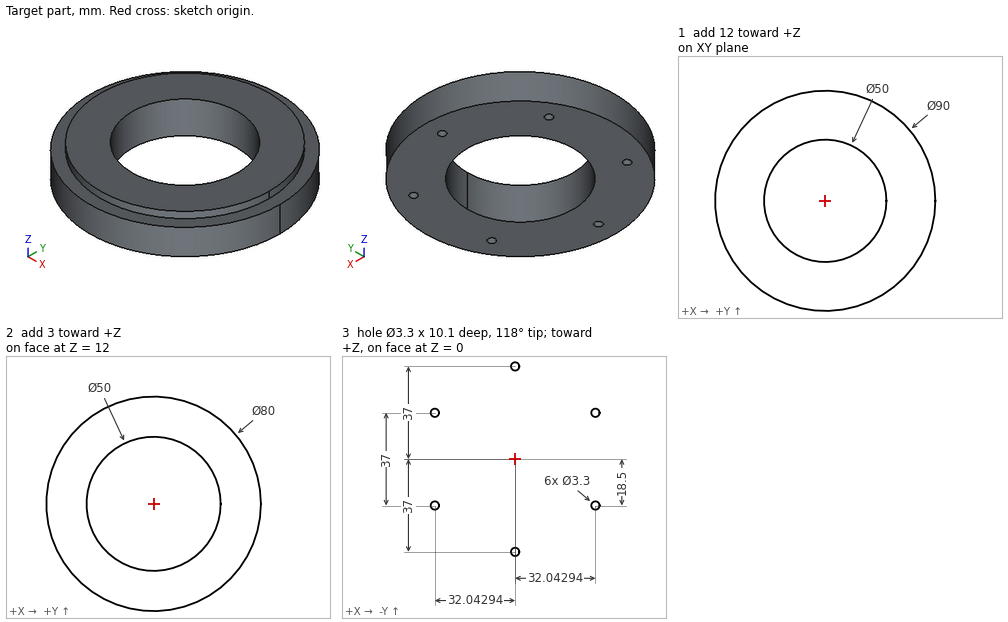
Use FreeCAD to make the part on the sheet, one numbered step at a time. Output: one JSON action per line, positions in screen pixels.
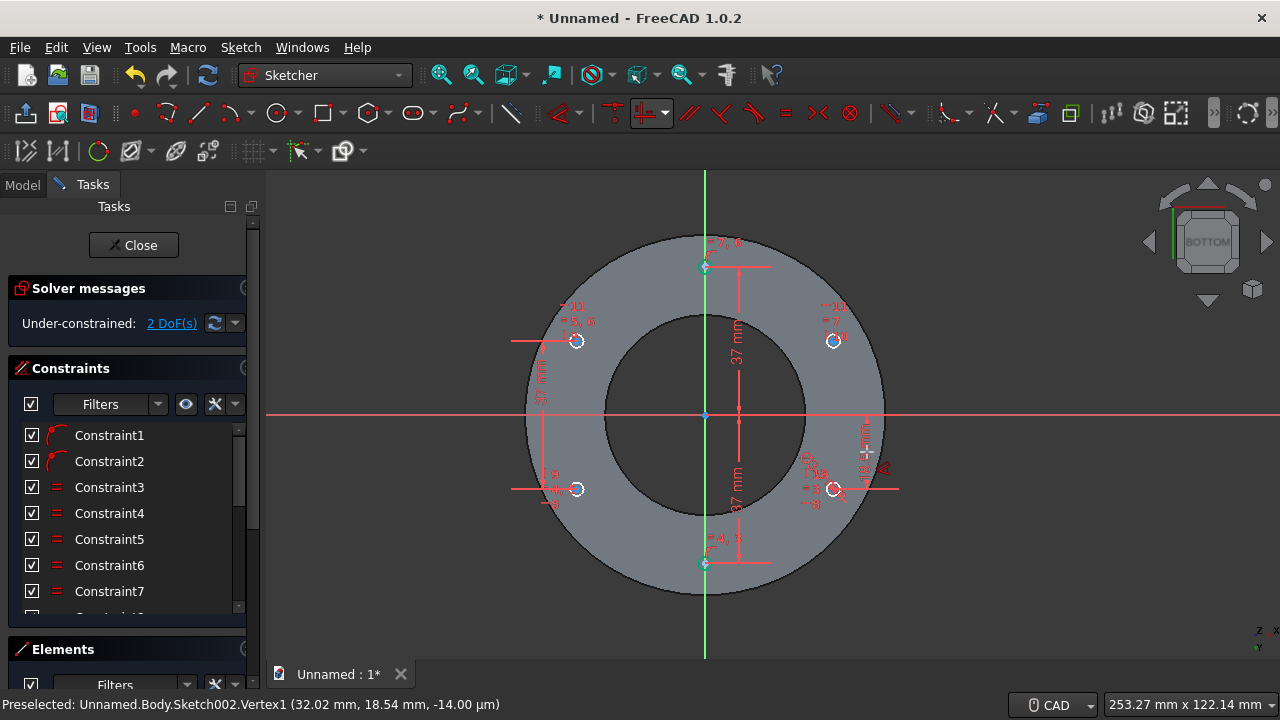
{"action": "left_click", "coordinate": [833, 489]}
{"action": "left_click", "coordinate": [769, 523]}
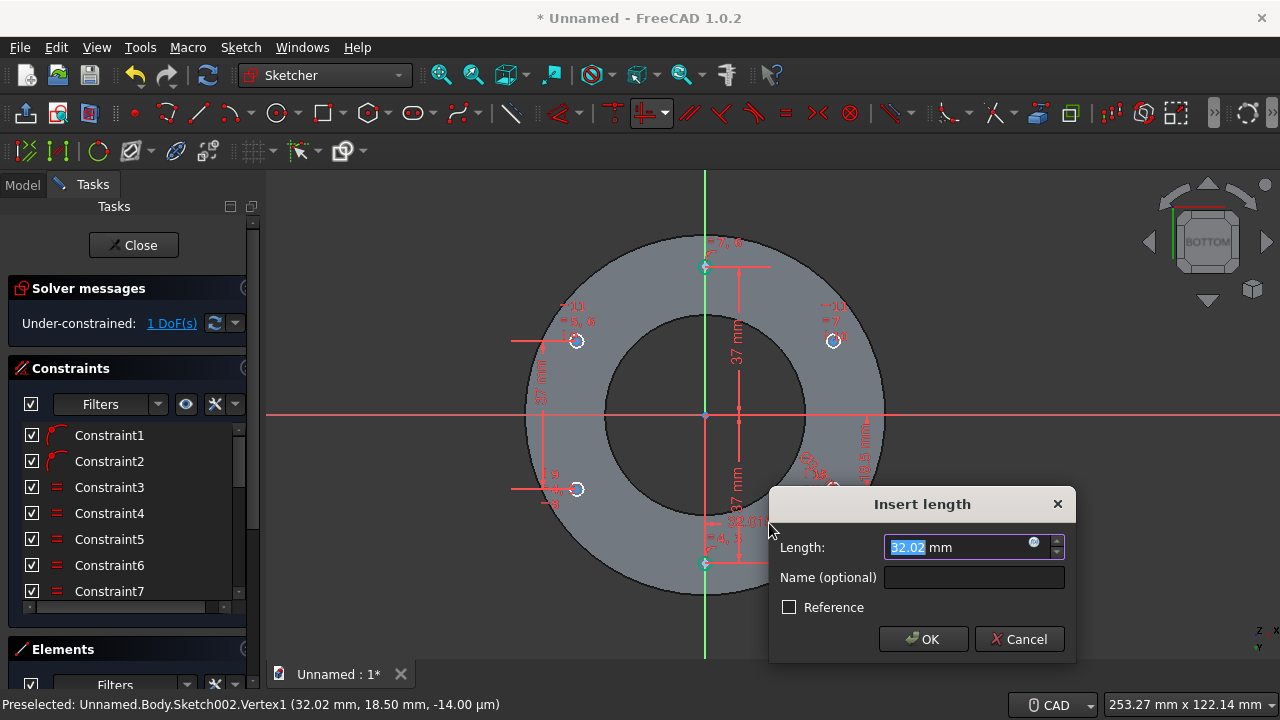
{"action": "type", "text": "32.04294"}
{"action": "key", "text": "Return"}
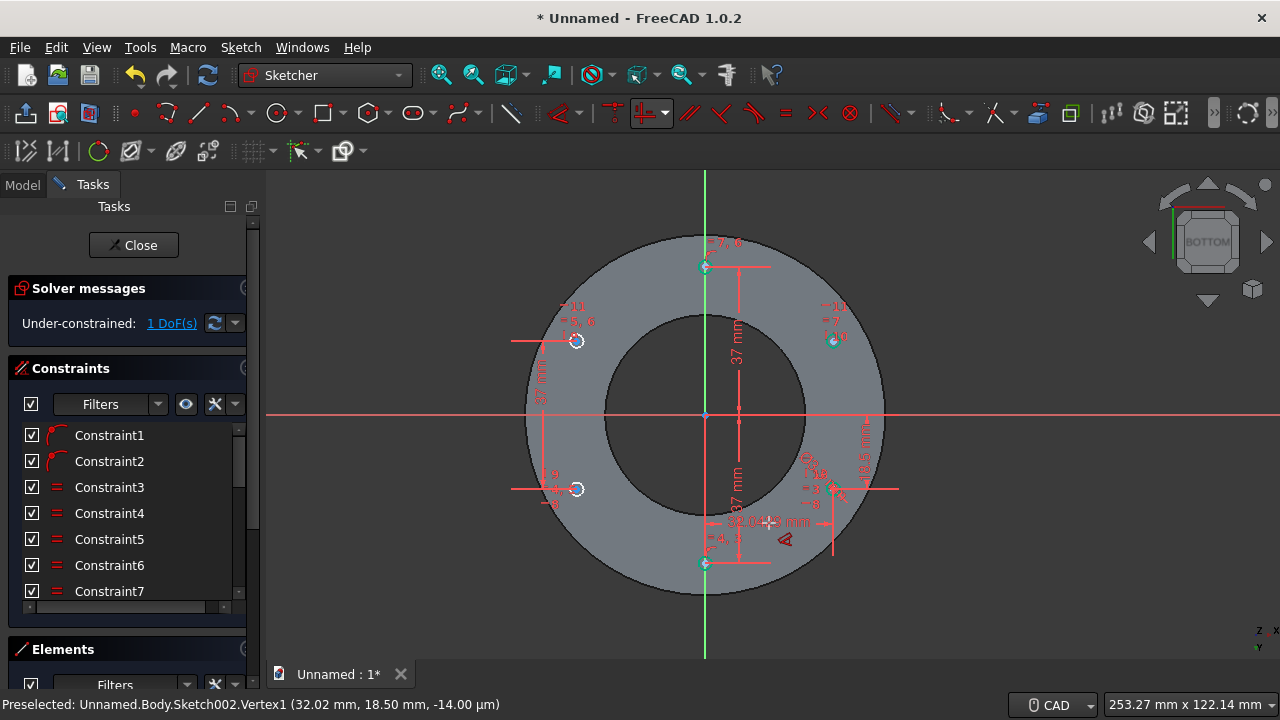
{"action": "left_click", "coordinate": [577, 489]}
{"action": "left_click", "coordinate": [641, 523]}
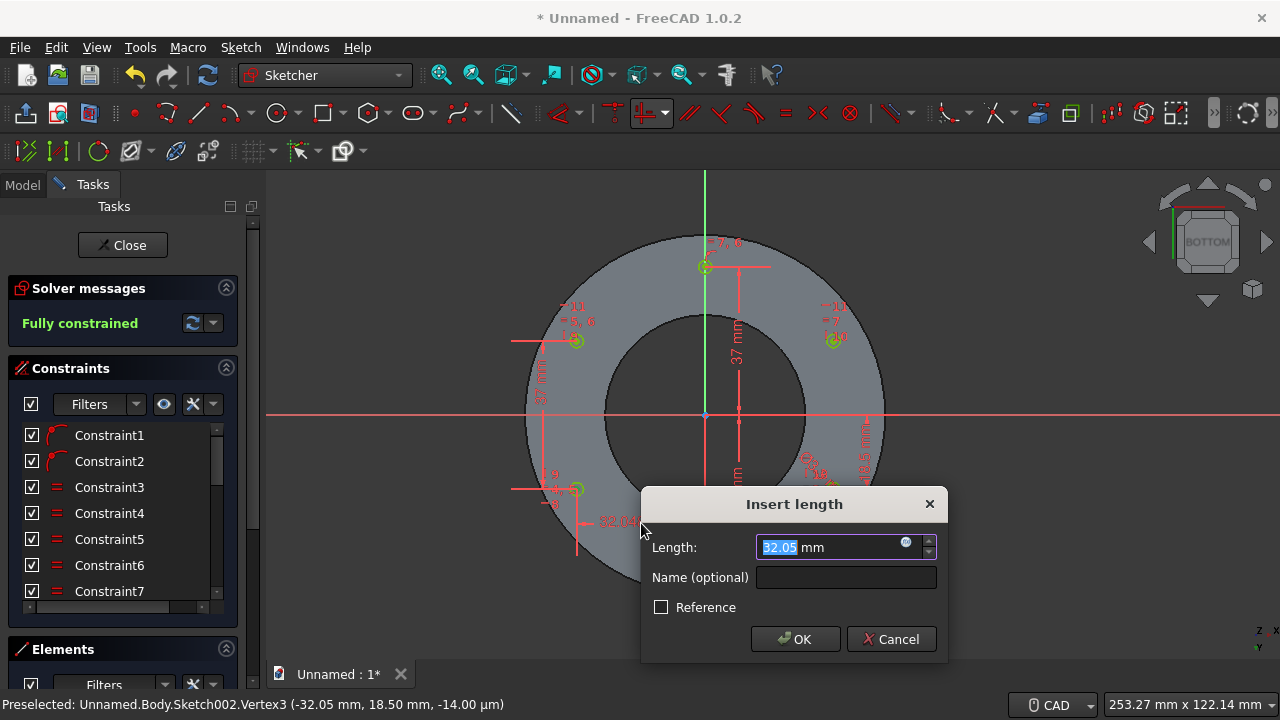
{"action": "type", "text": "32.04294"}
{"action": "key", "text": "Return"}
{"action": "key", "text": "Escape"}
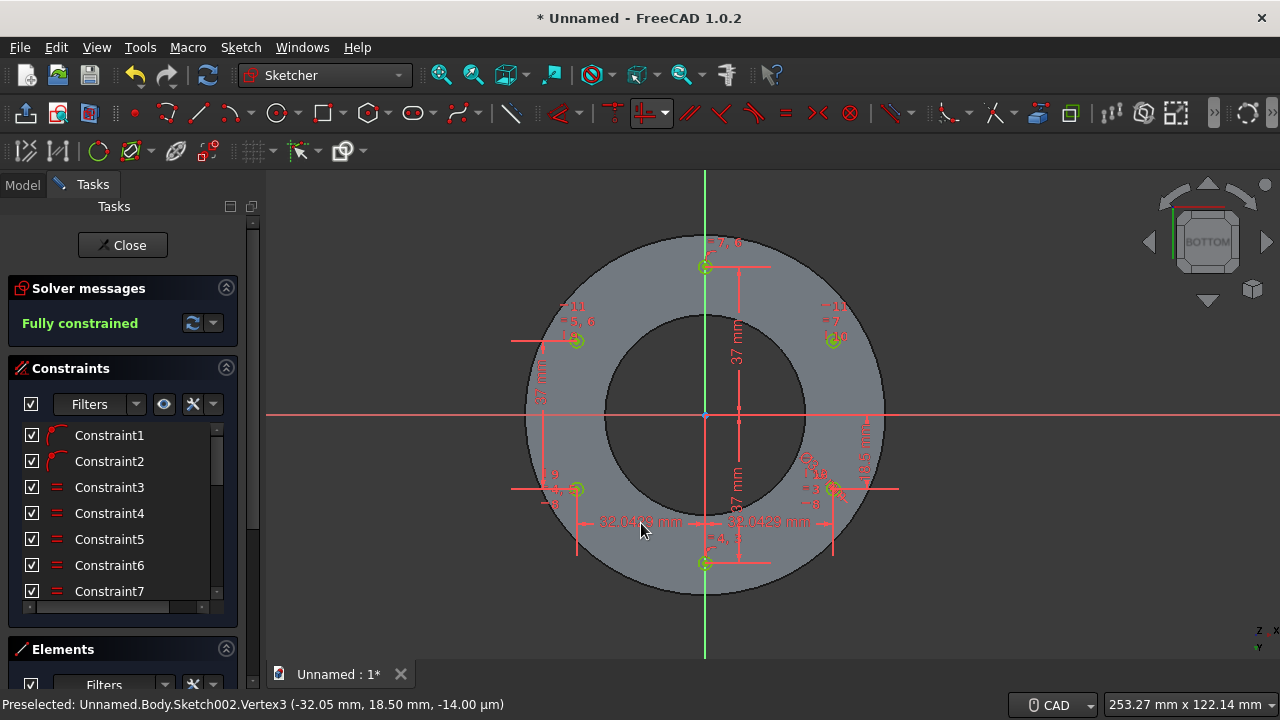
{"action": "left_click", "coordinate": [123, 245]}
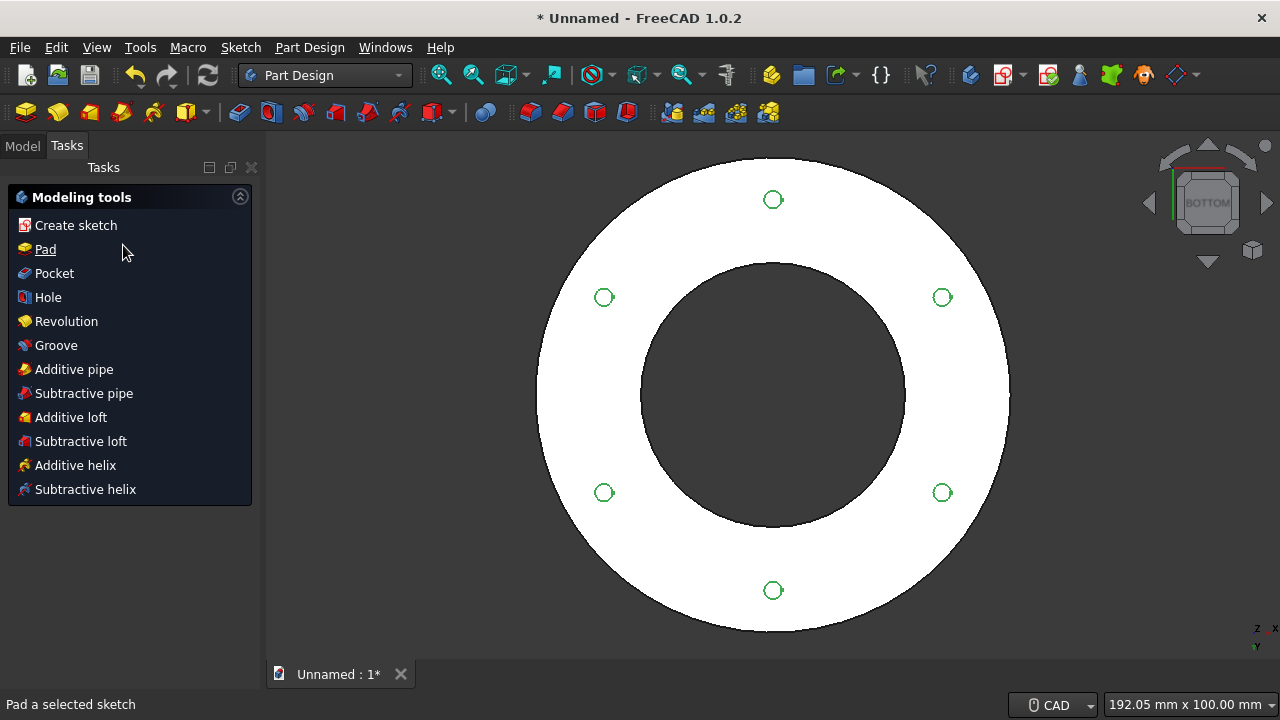
{"action": "left_click", "coordinate": [272, 112]}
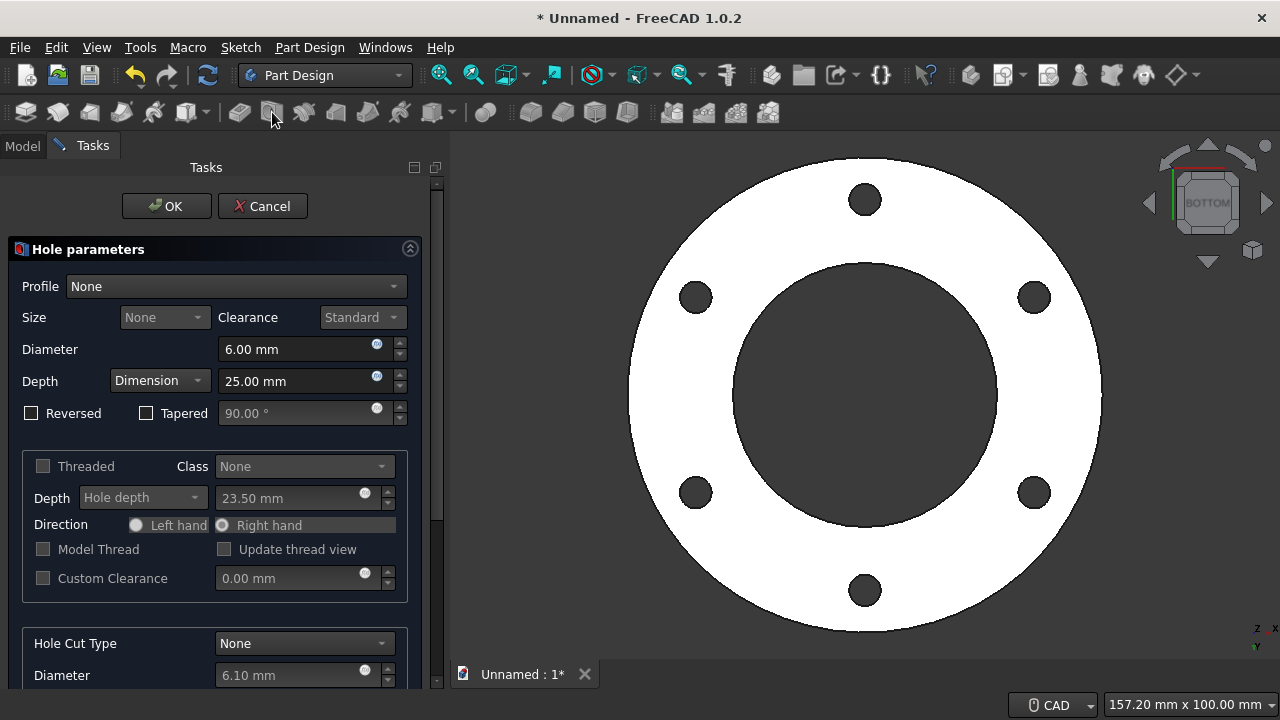
{"action": "triple_click", "coordinate": [305, 349]}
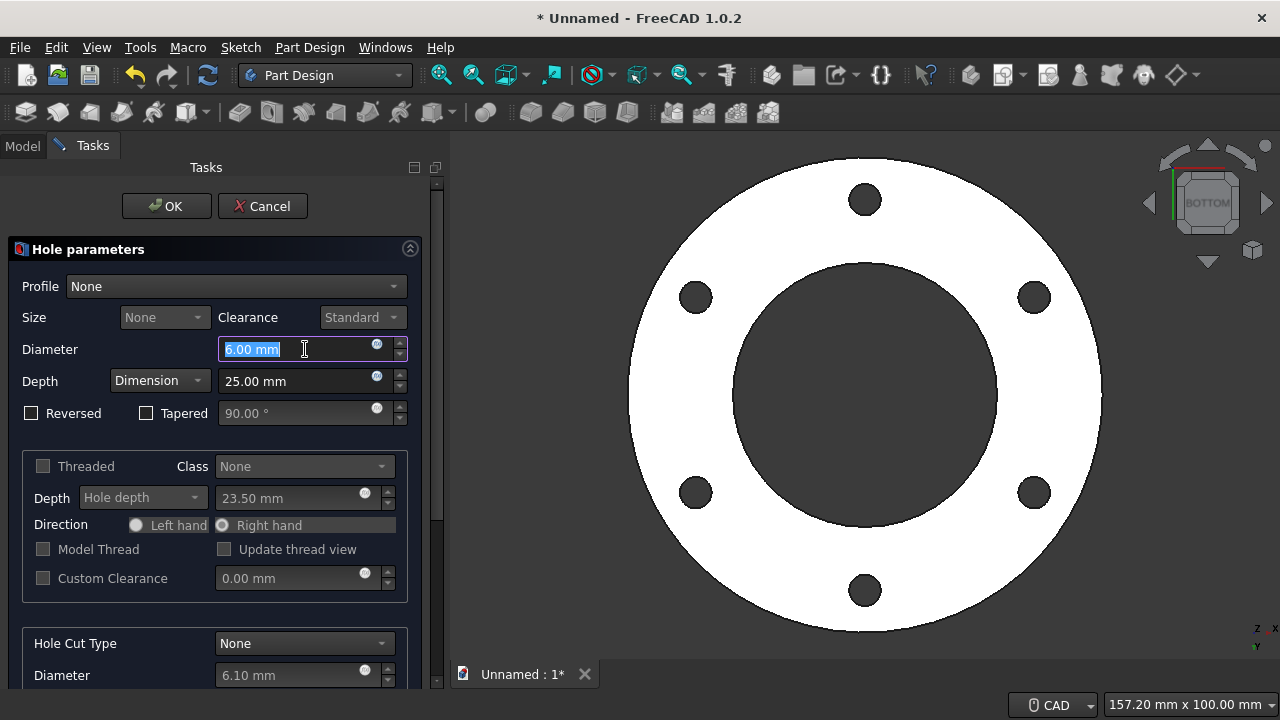
{"action": "type", "text": "3.3"}
{"action": "key", "text": "Tab"}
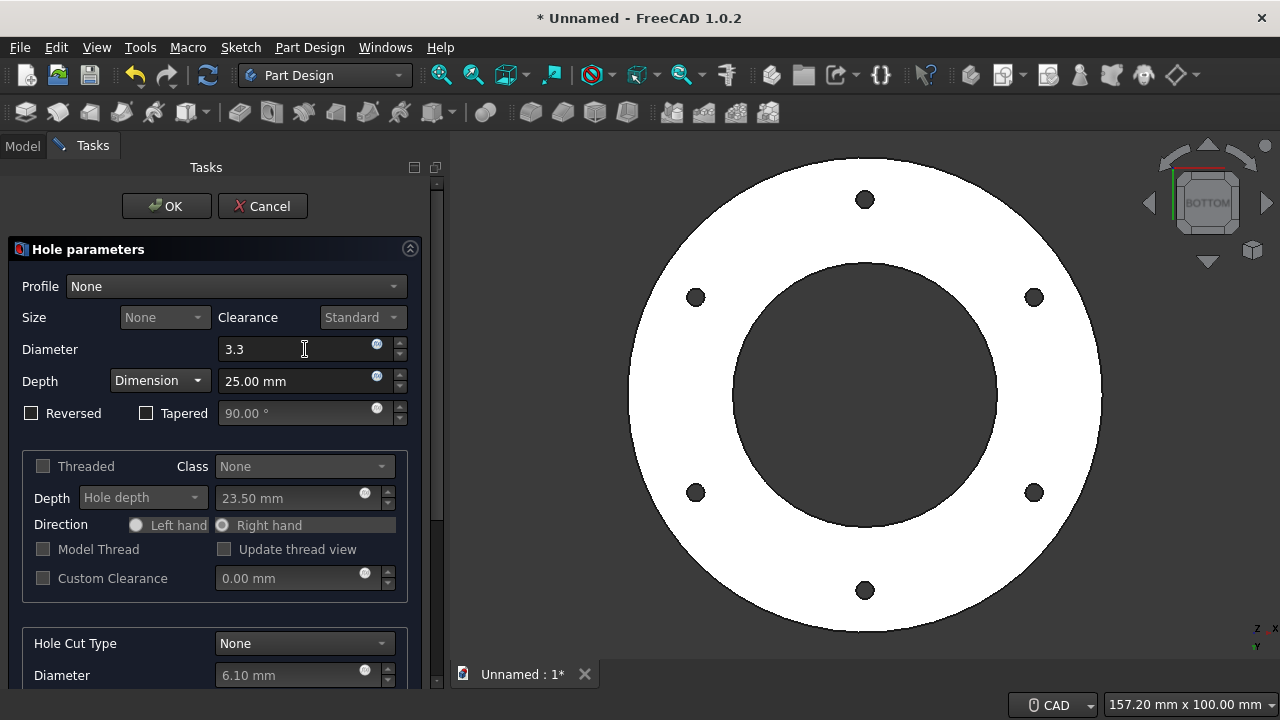
{"action": "triple_click", "coordinate": [305, 381]}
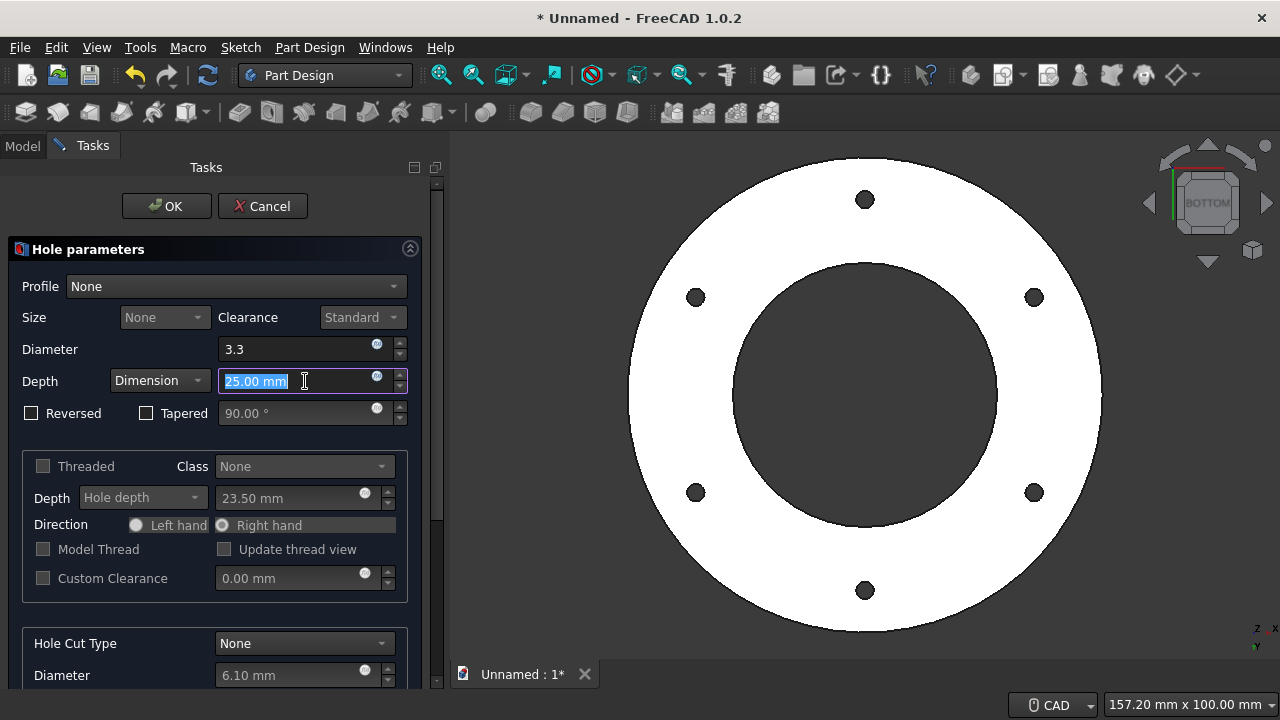
{"action": "type", "text": "10.1"}
{"action": "key", "text": "Tab"}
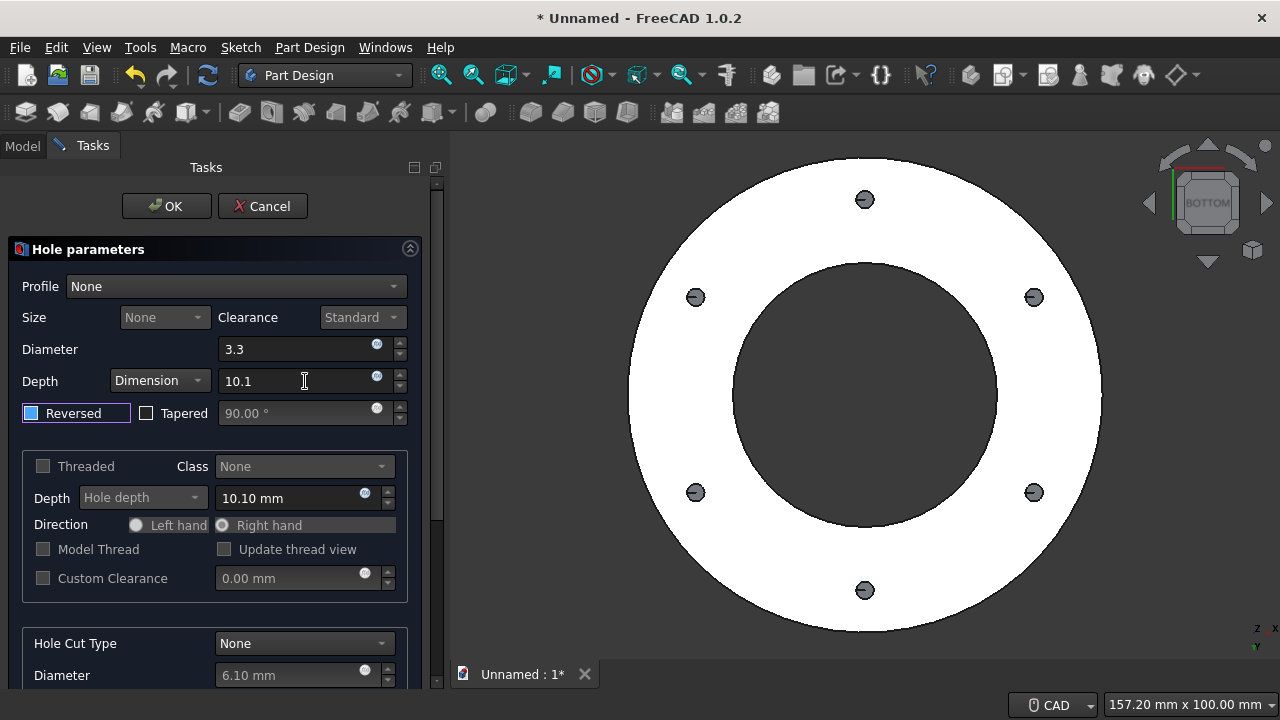
{"action": "left_click", "coordinate": [167, 206]}